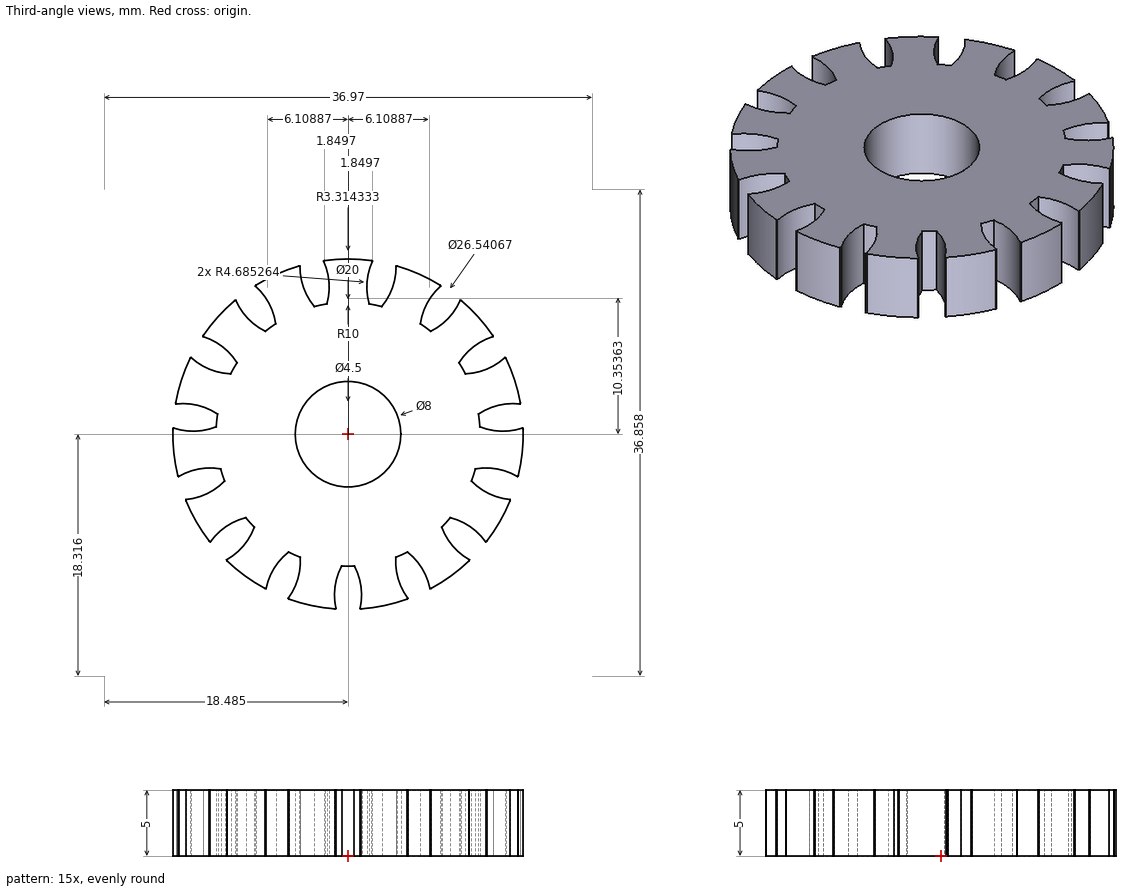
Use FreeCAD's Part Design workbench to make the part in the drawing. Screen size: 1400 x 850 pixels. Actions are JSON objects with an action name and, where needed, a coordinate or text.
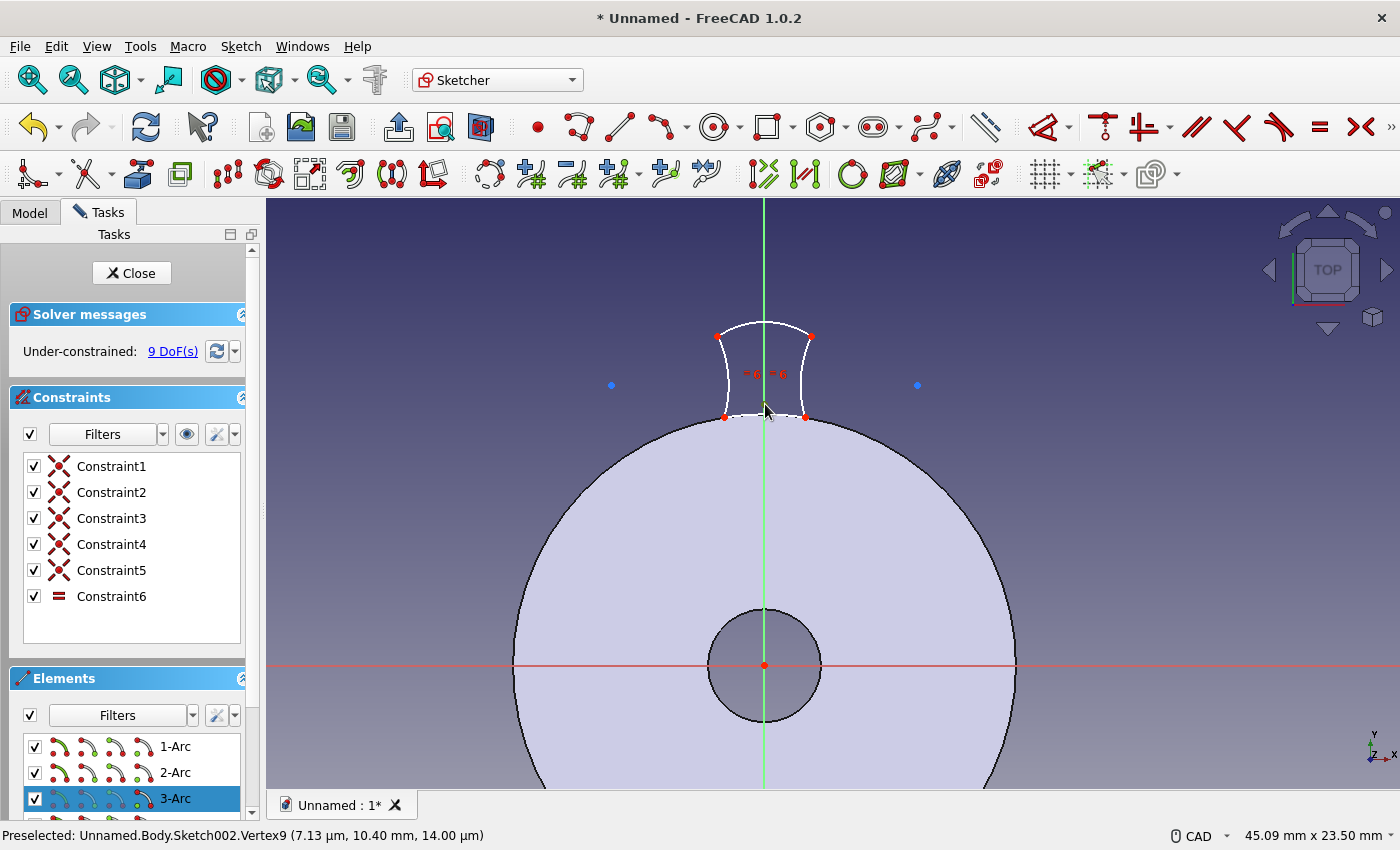
{"action": "left_click", "coordinate": [764, 723]}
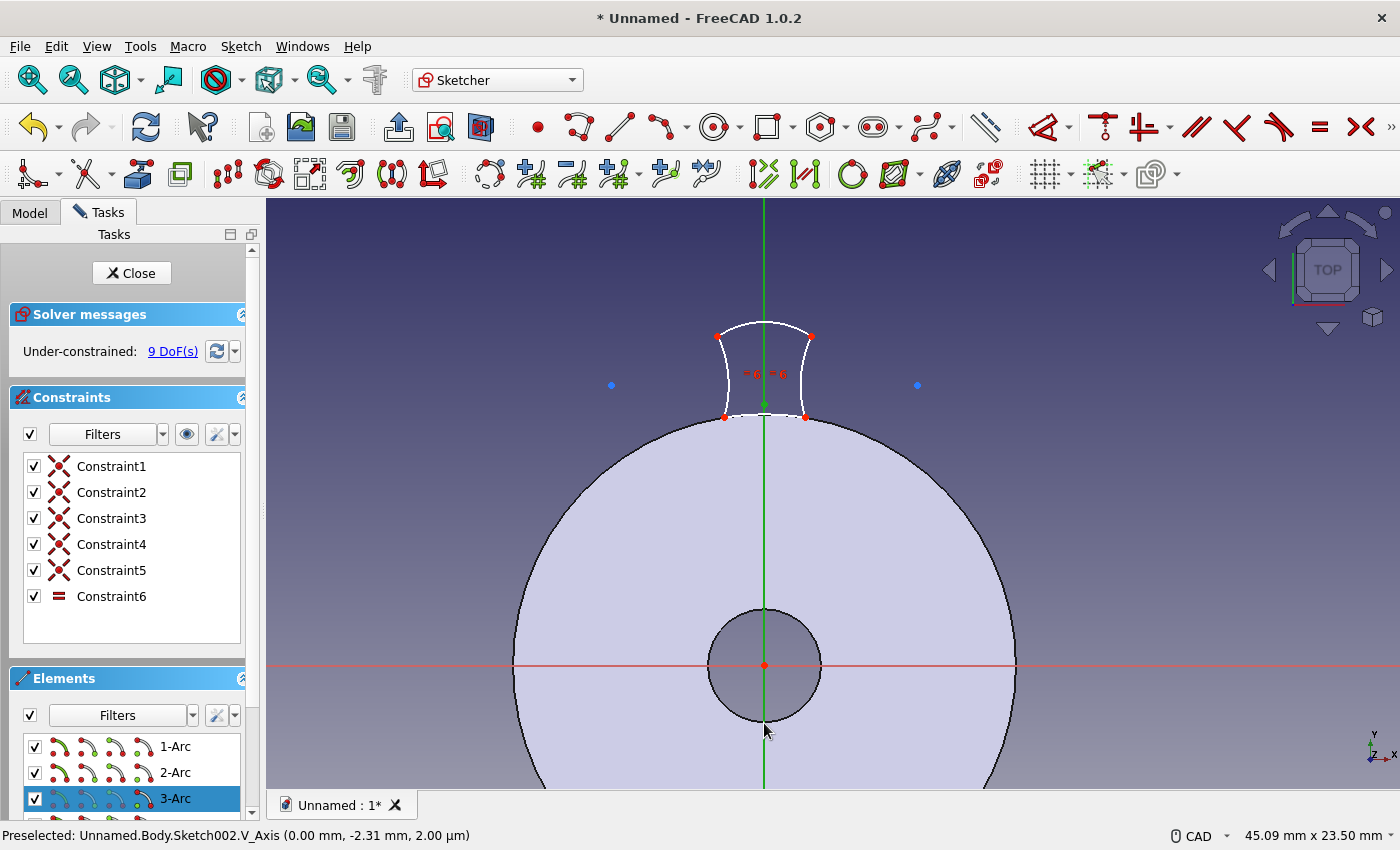
{"action": "key", "text": "c"}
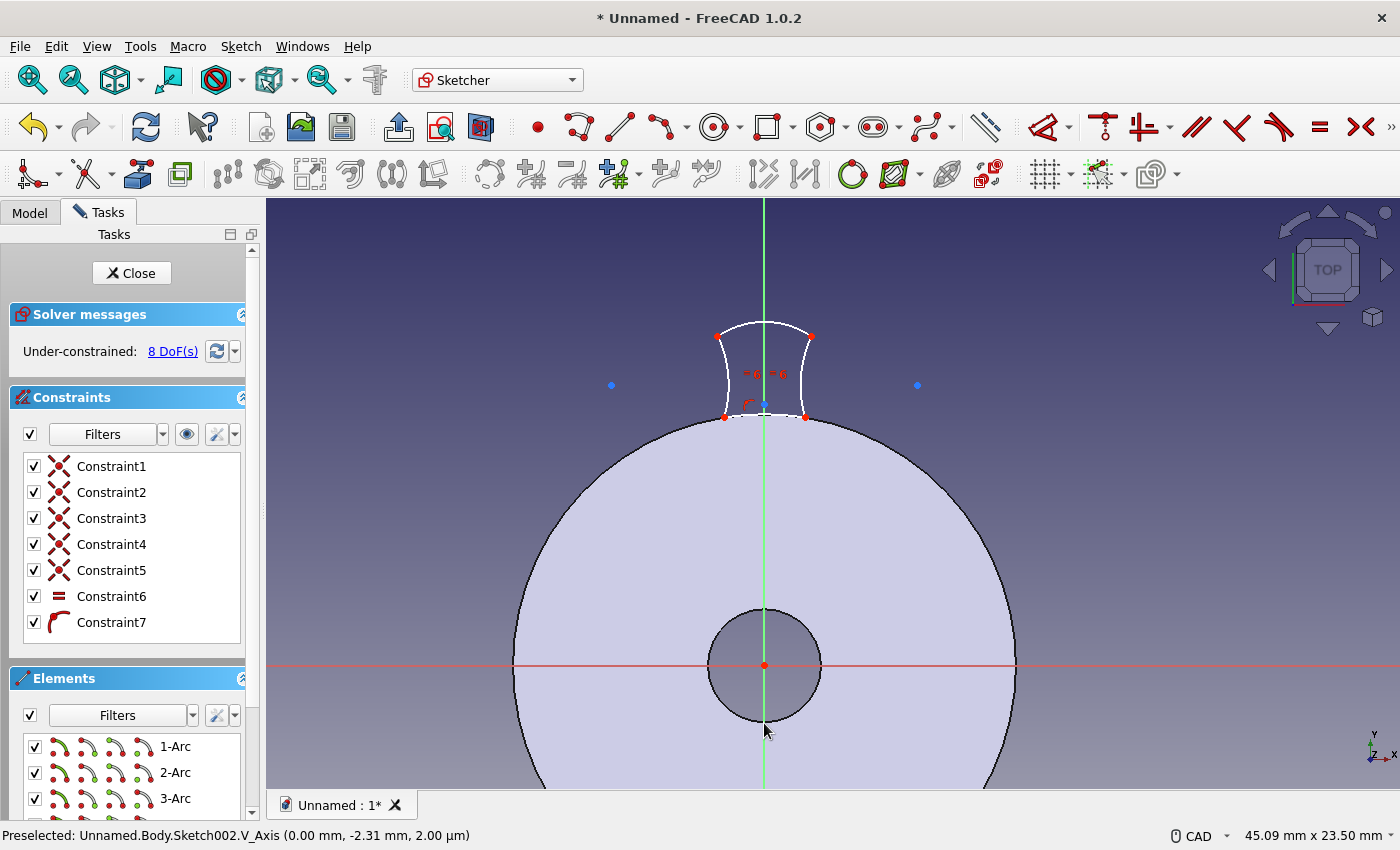
{"action": "left_click", "coordinate": [1042, 128]}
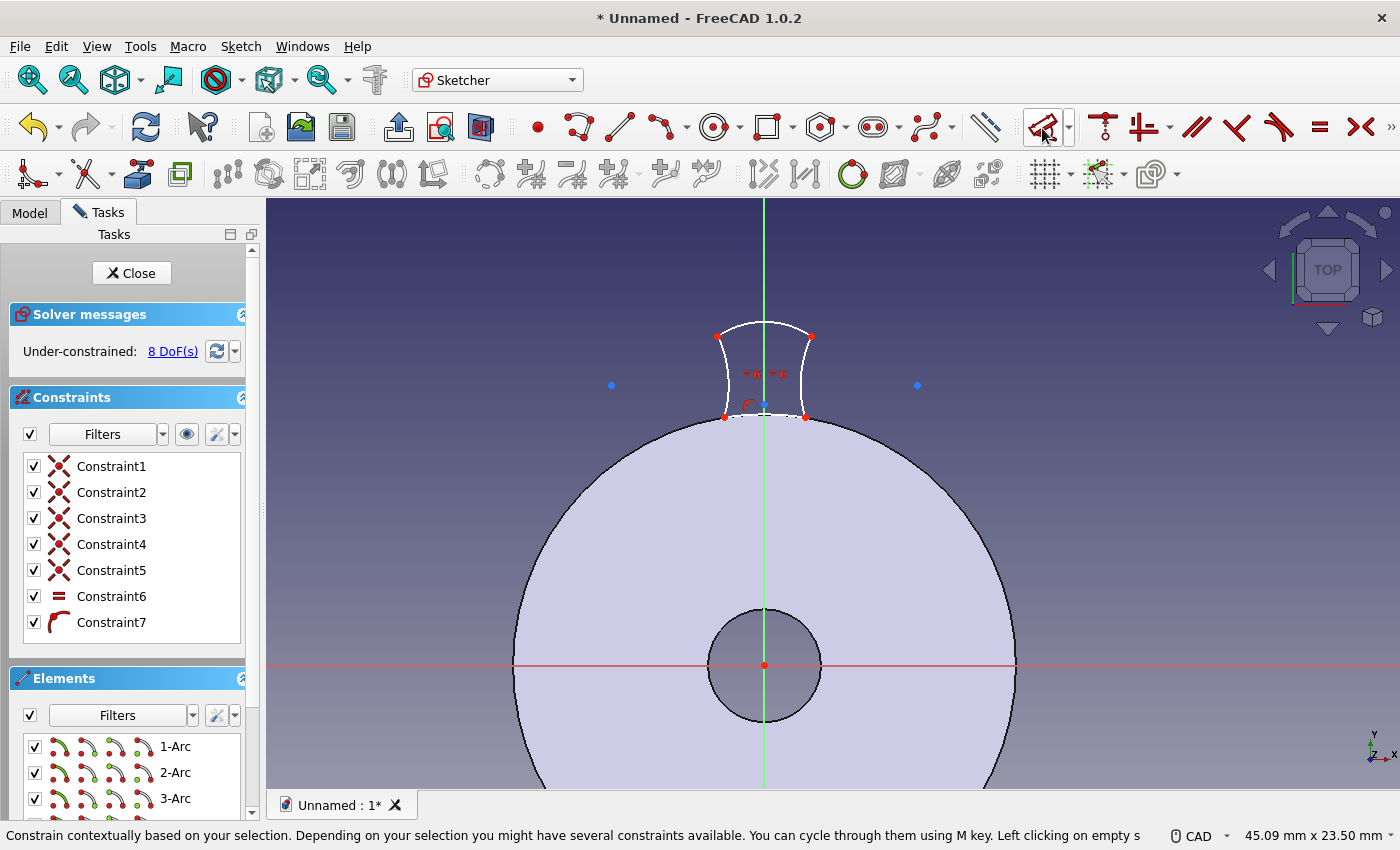
{"action": "left_click", "coordinate": [781, 415]}
{"action": "left_click", "coordinate": [783, 383]}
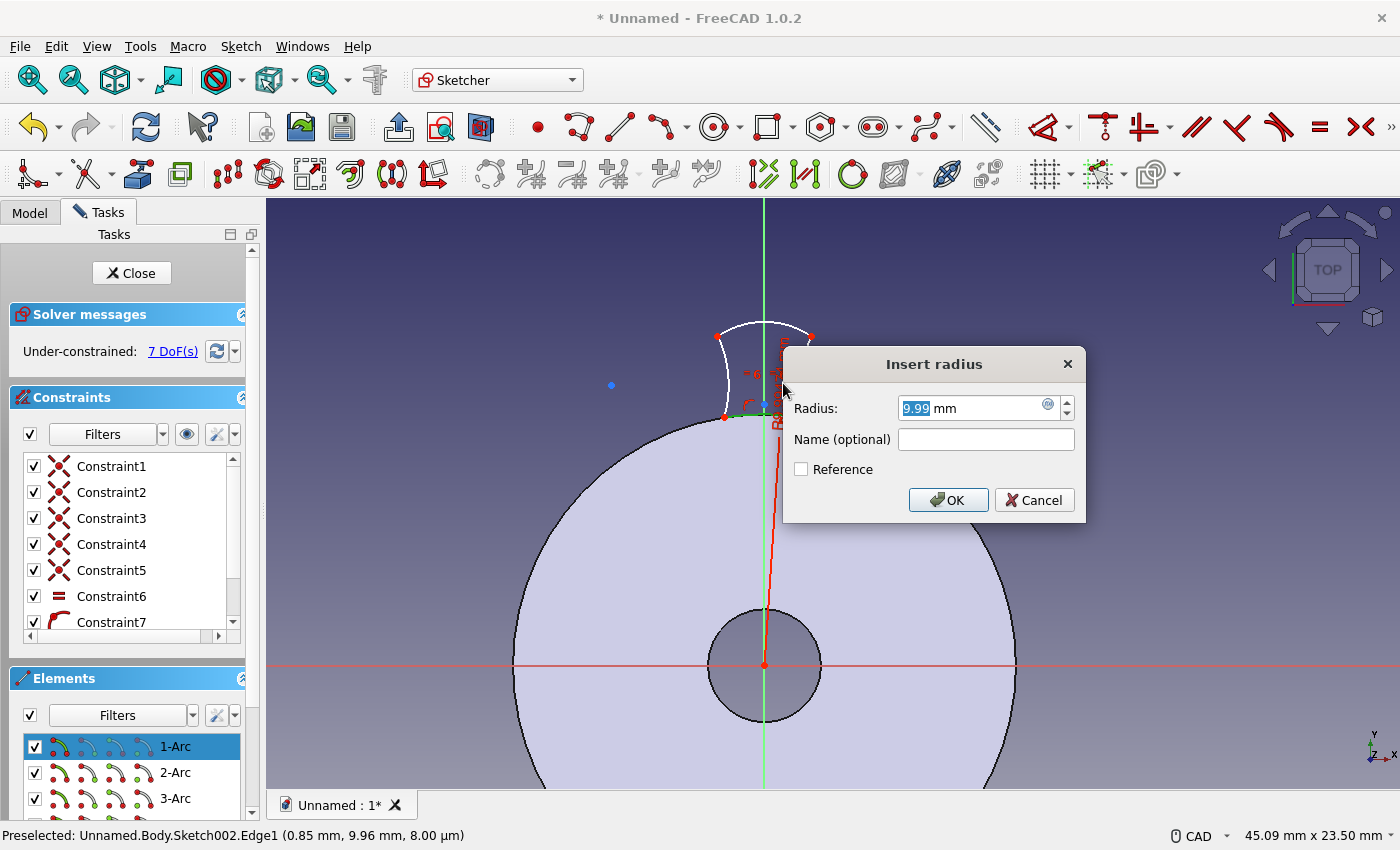
{"action": "type", "text": "10"}
{"action": "key", "text": "Return"}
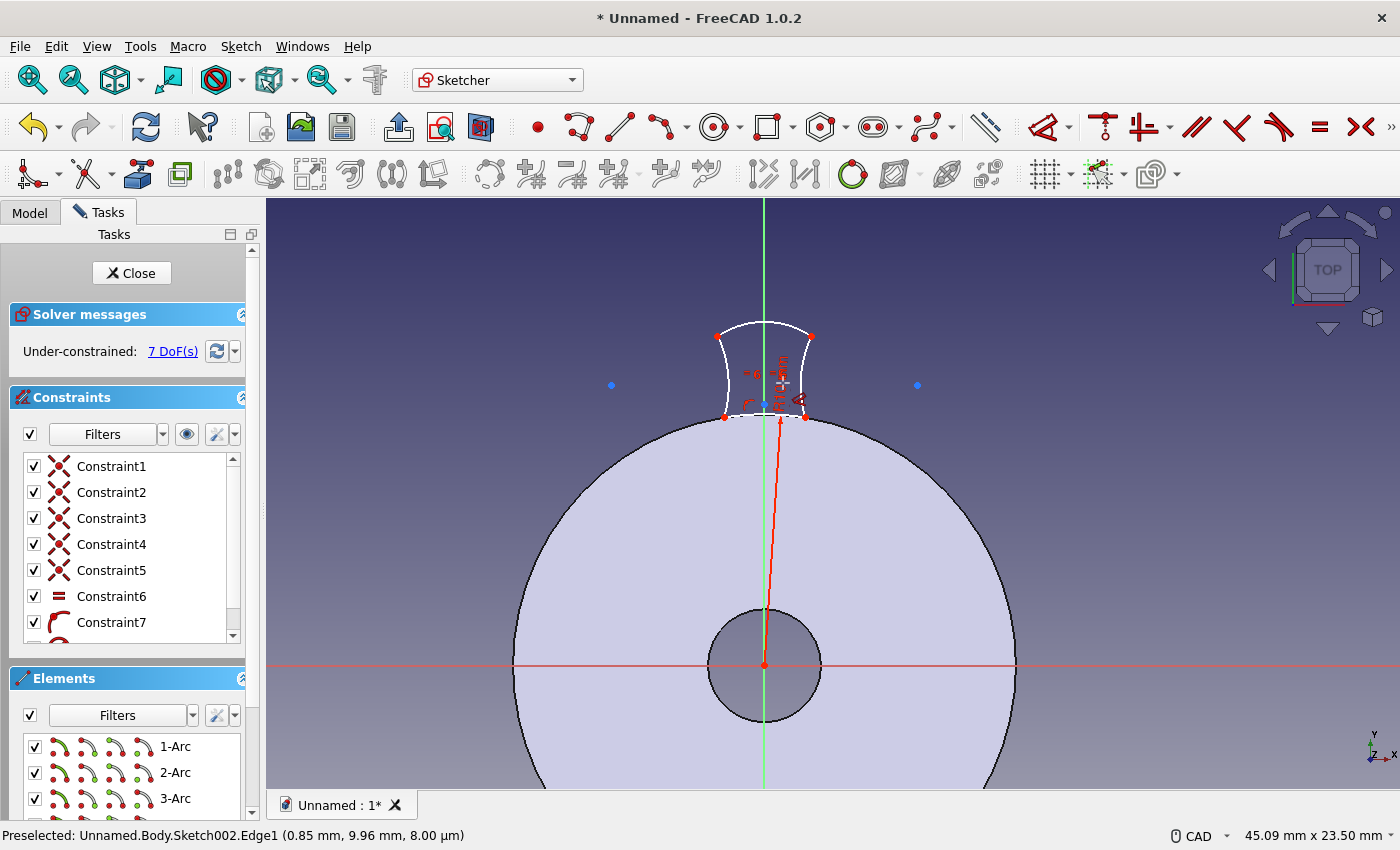
{"action": "left_click", "coordinate": [803, 360]}
{"action": "left_click", "coordinate": [805, 287]}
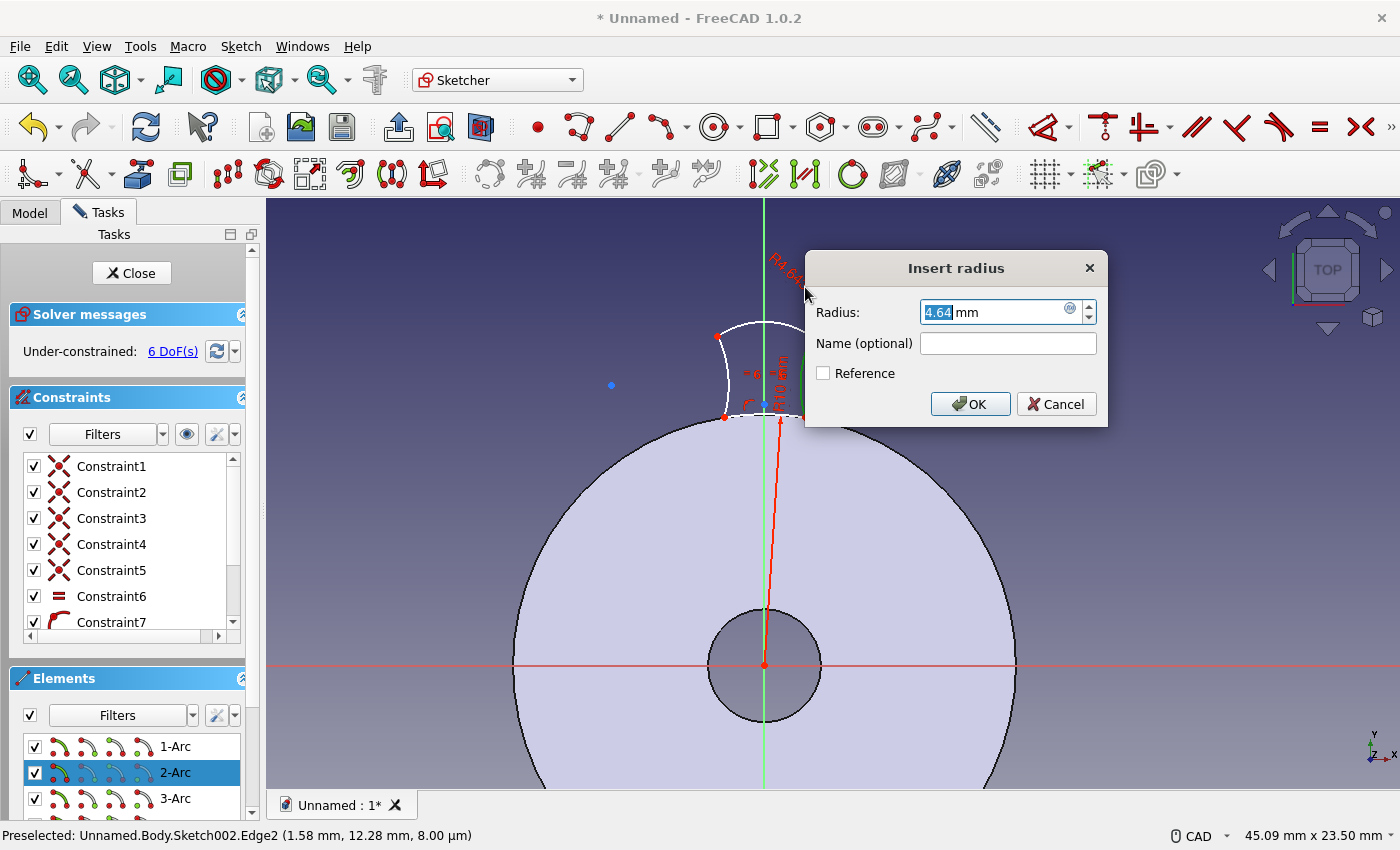
{"action": "type", "text": "4.685264"}
{"action": "key", "text": "Return"}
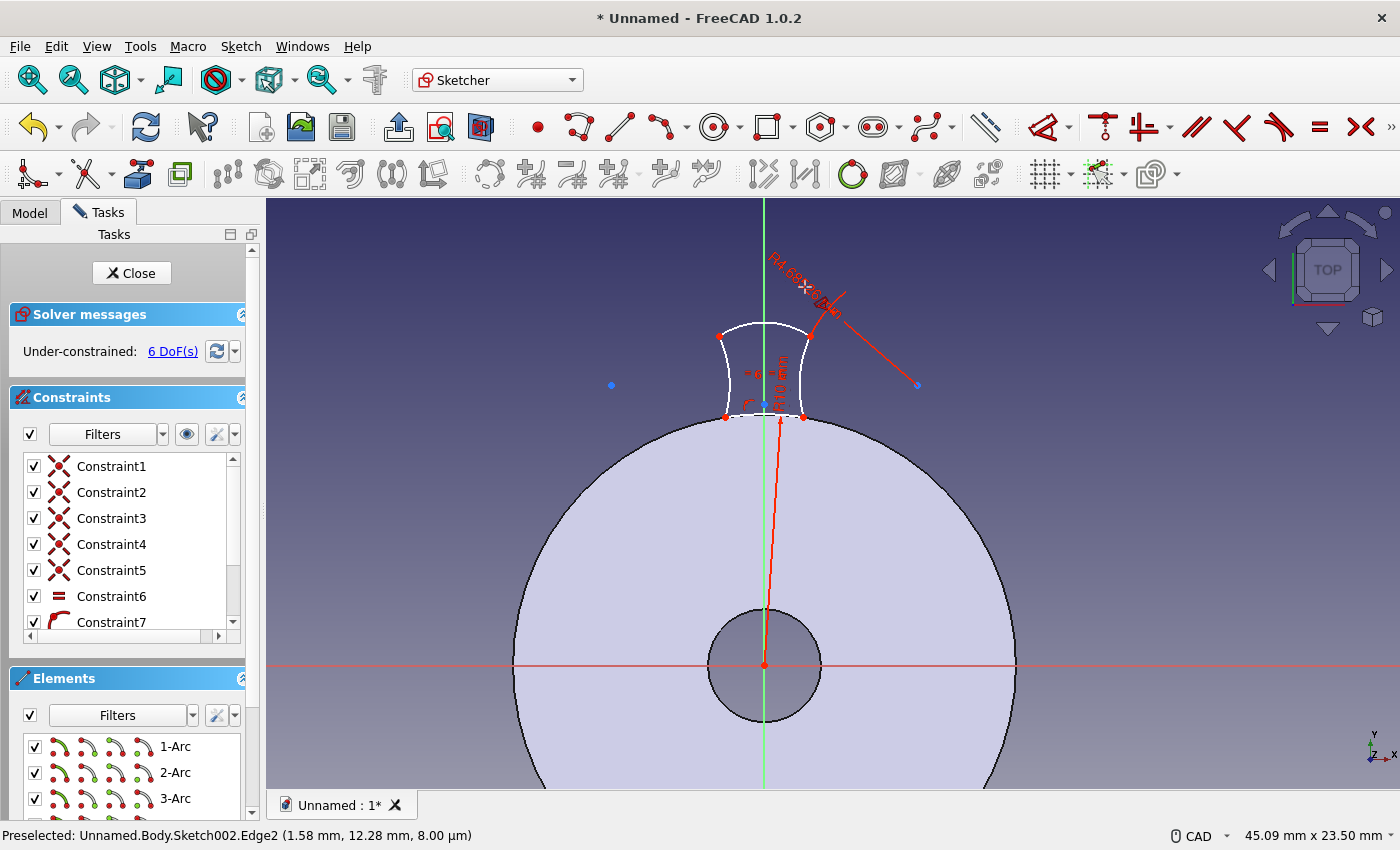
{"action": "left_click", "coordinate": [784, 325]}
{"action": "left_click", "coordinate": [841, 320]}